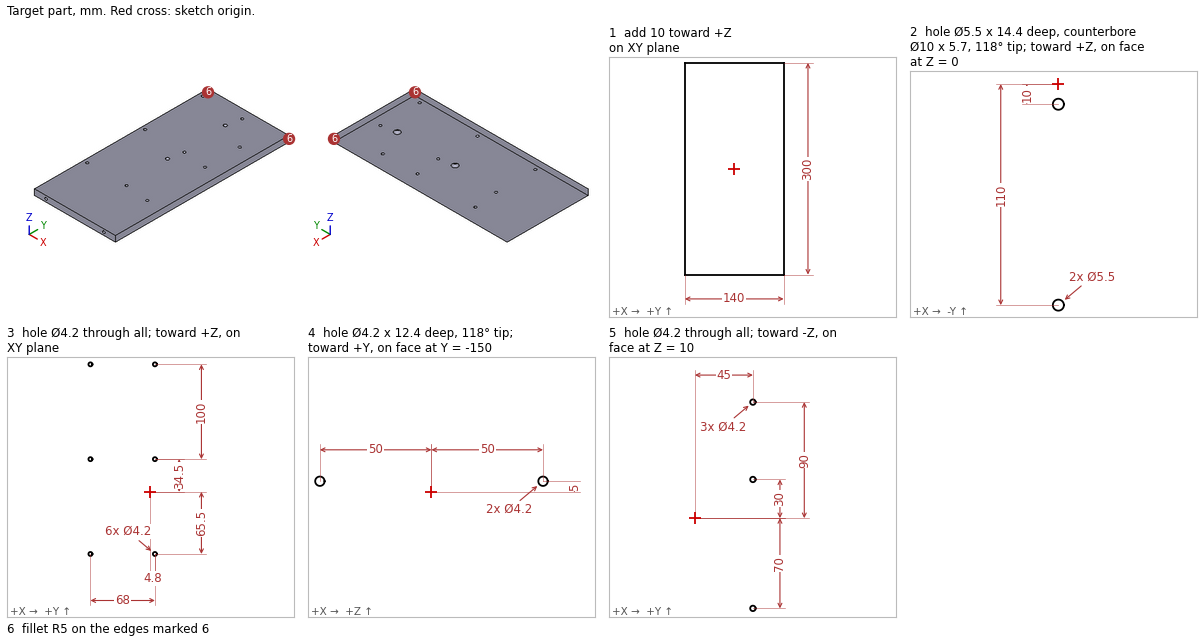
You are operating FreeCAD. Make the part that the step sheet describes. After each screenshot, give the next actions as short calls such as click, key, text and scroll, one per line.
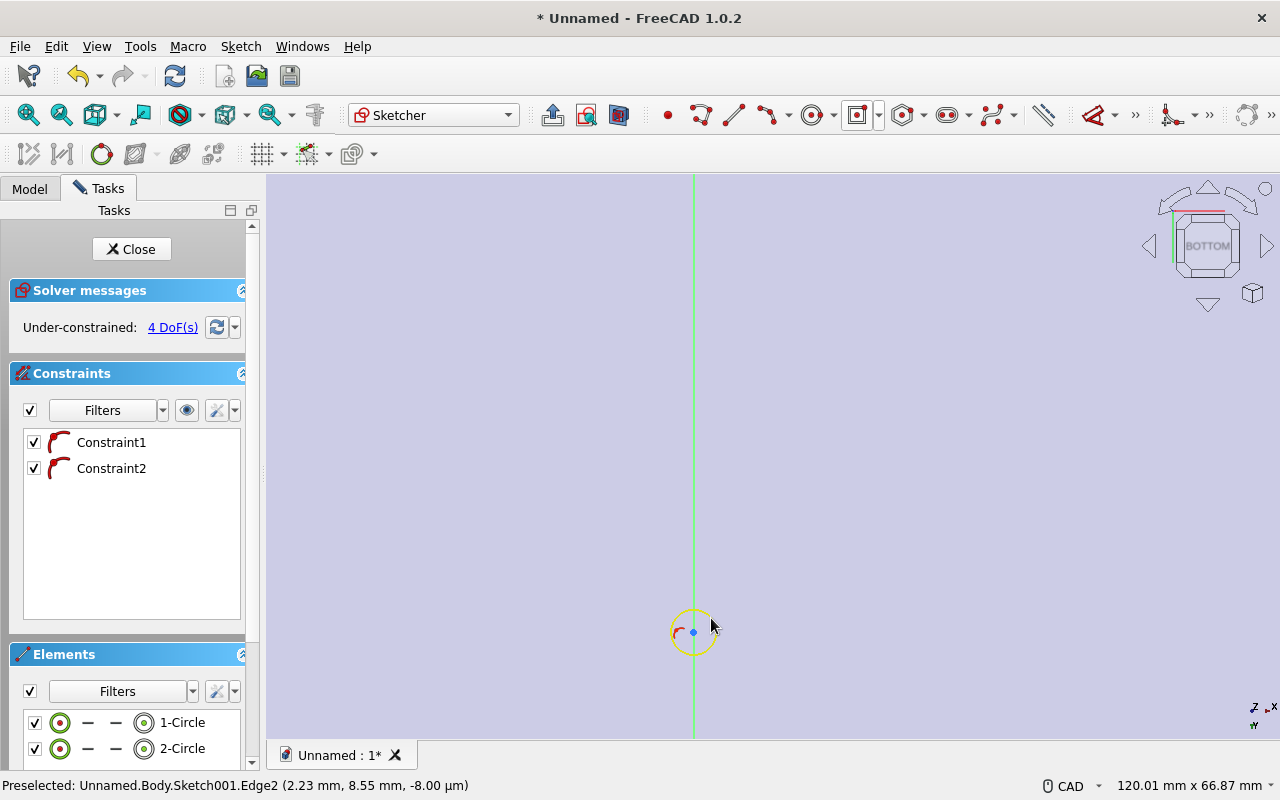
click(710, 616)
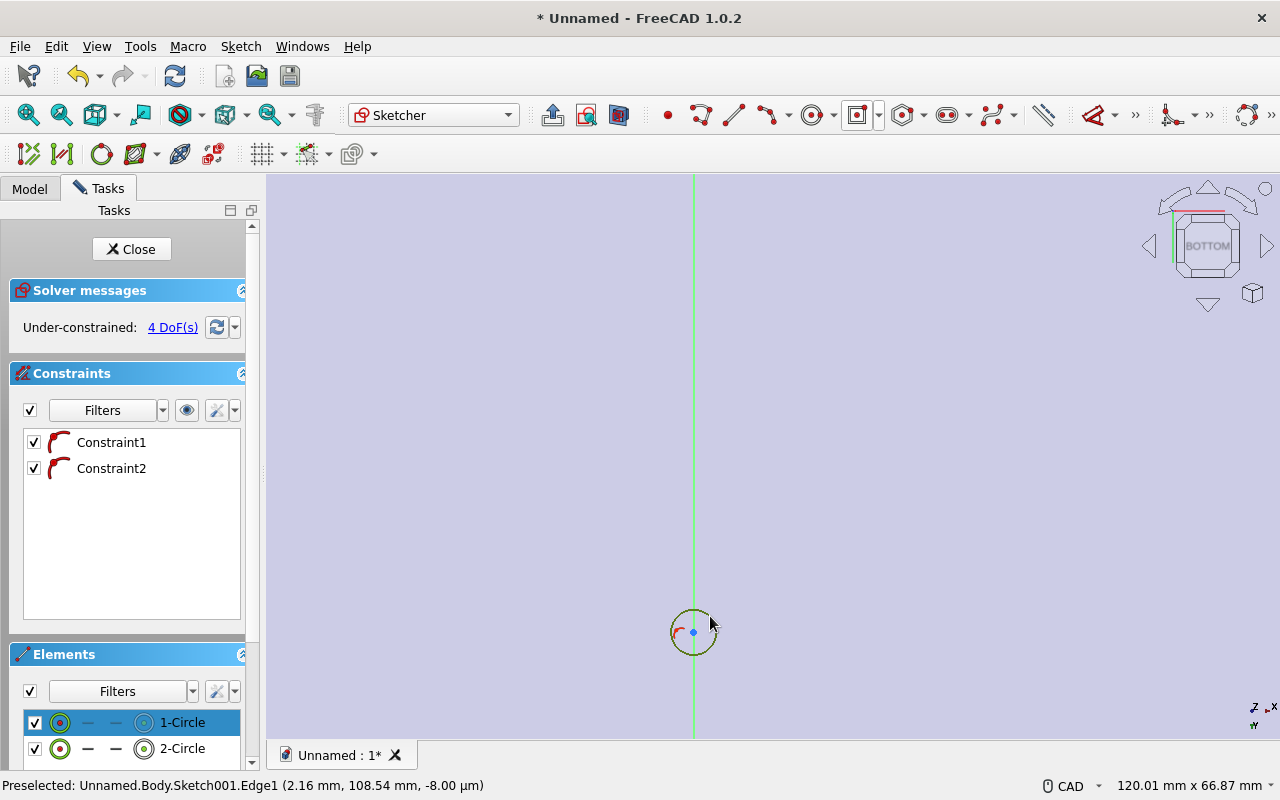
scroll(711, 618, down, 5)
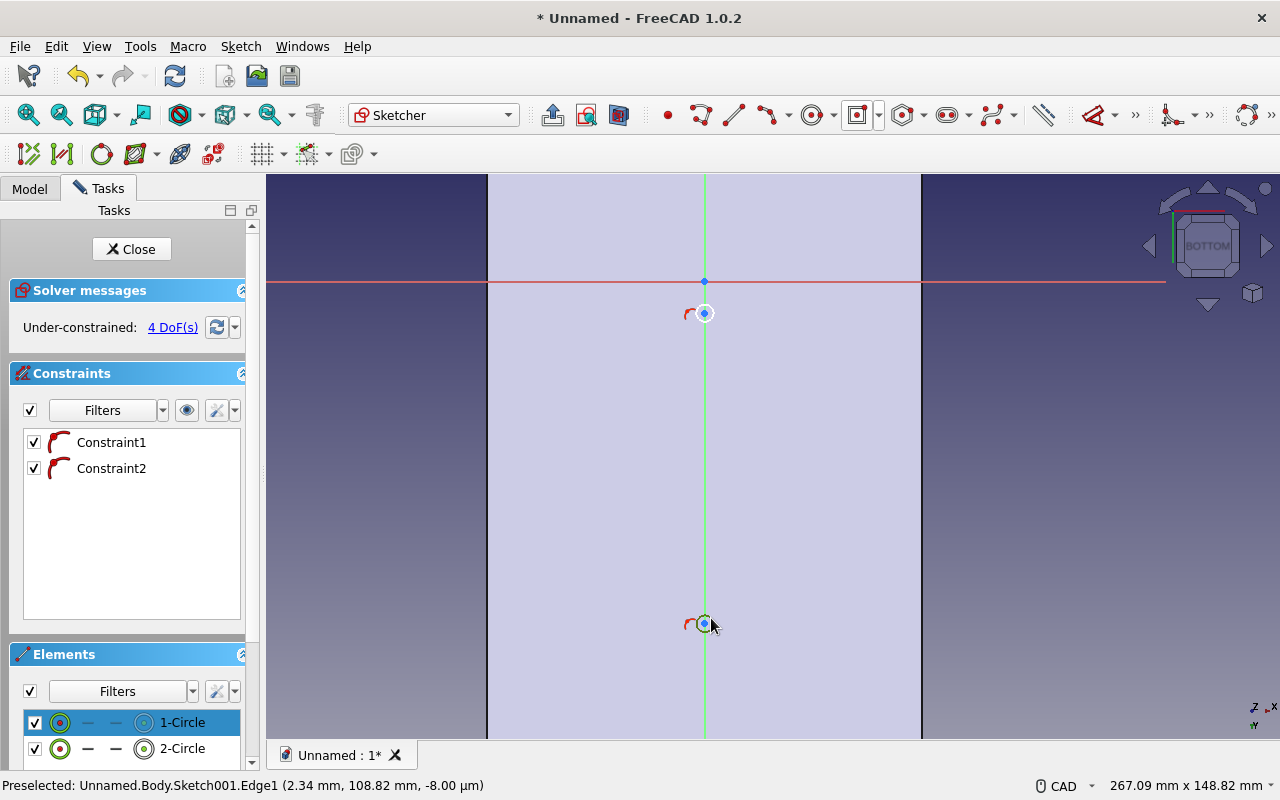
scroll(711, 307, up, 5)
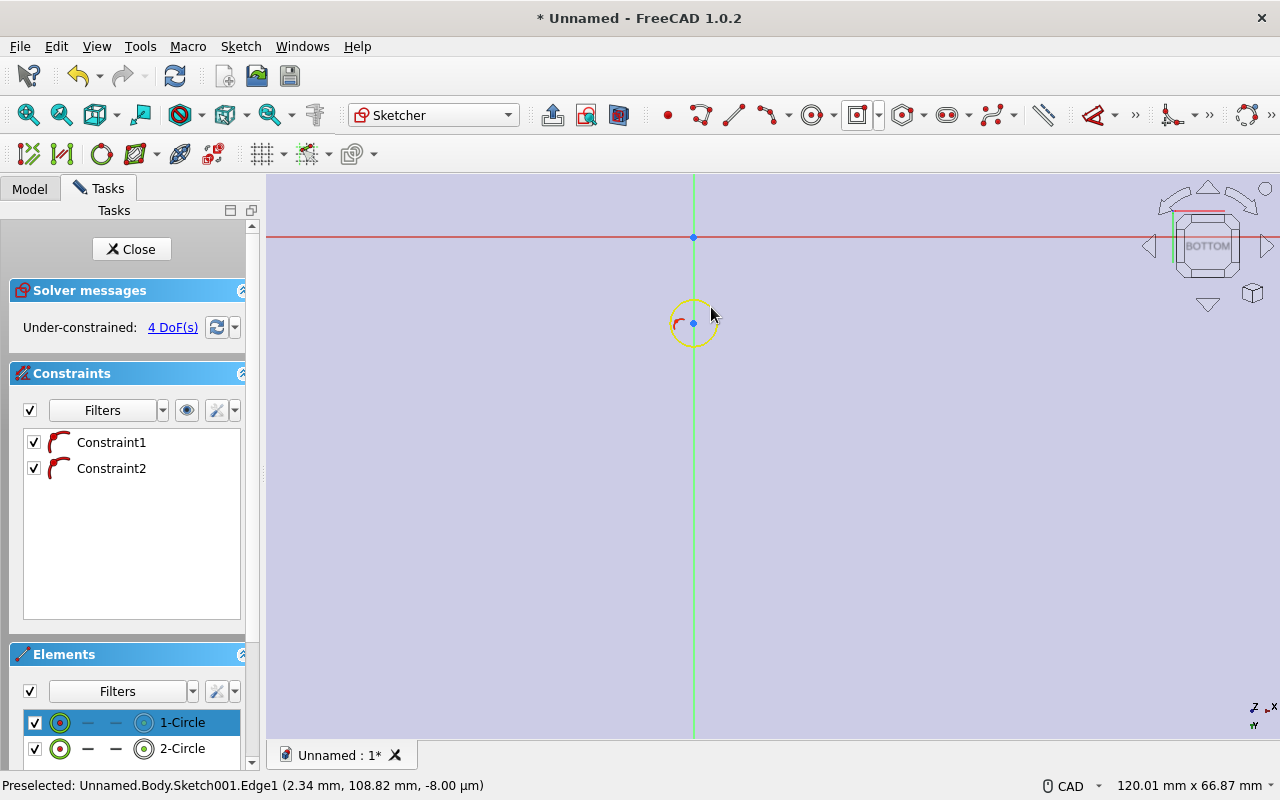
click(710, 307)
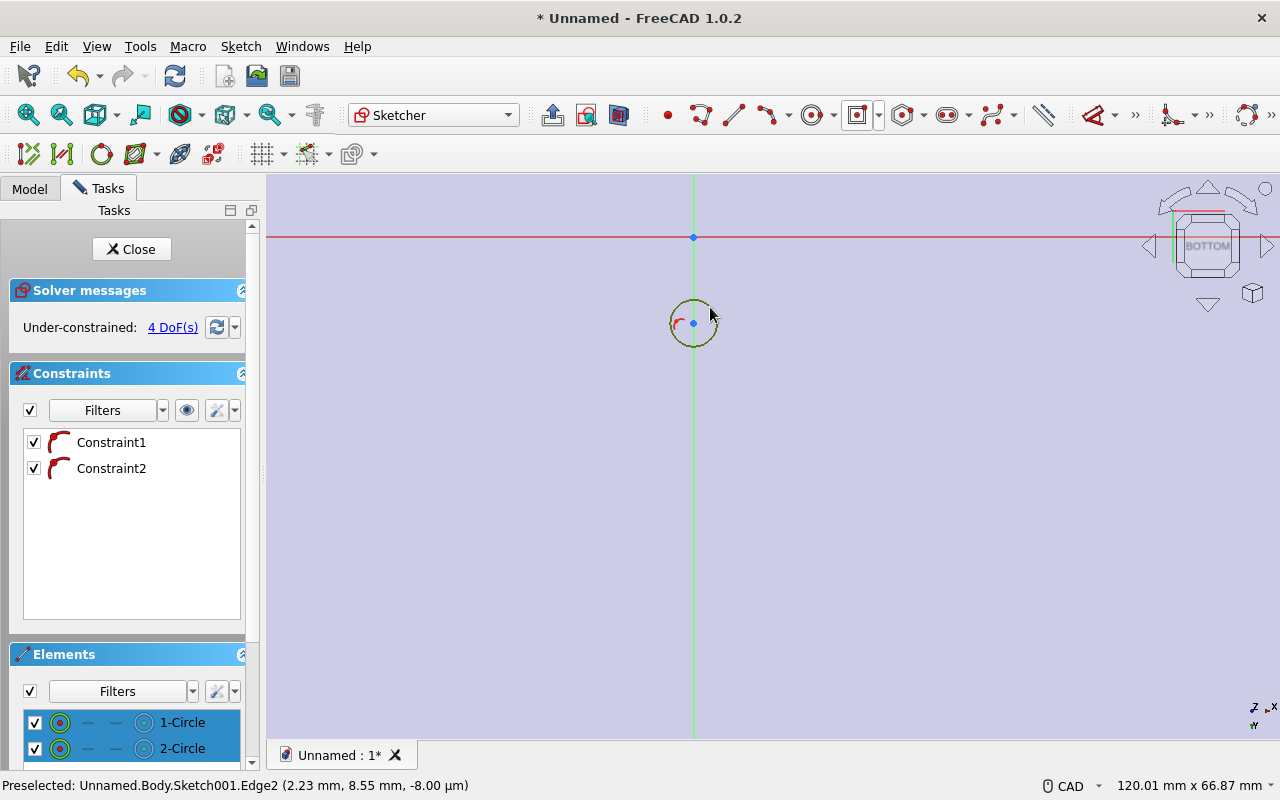
key(e)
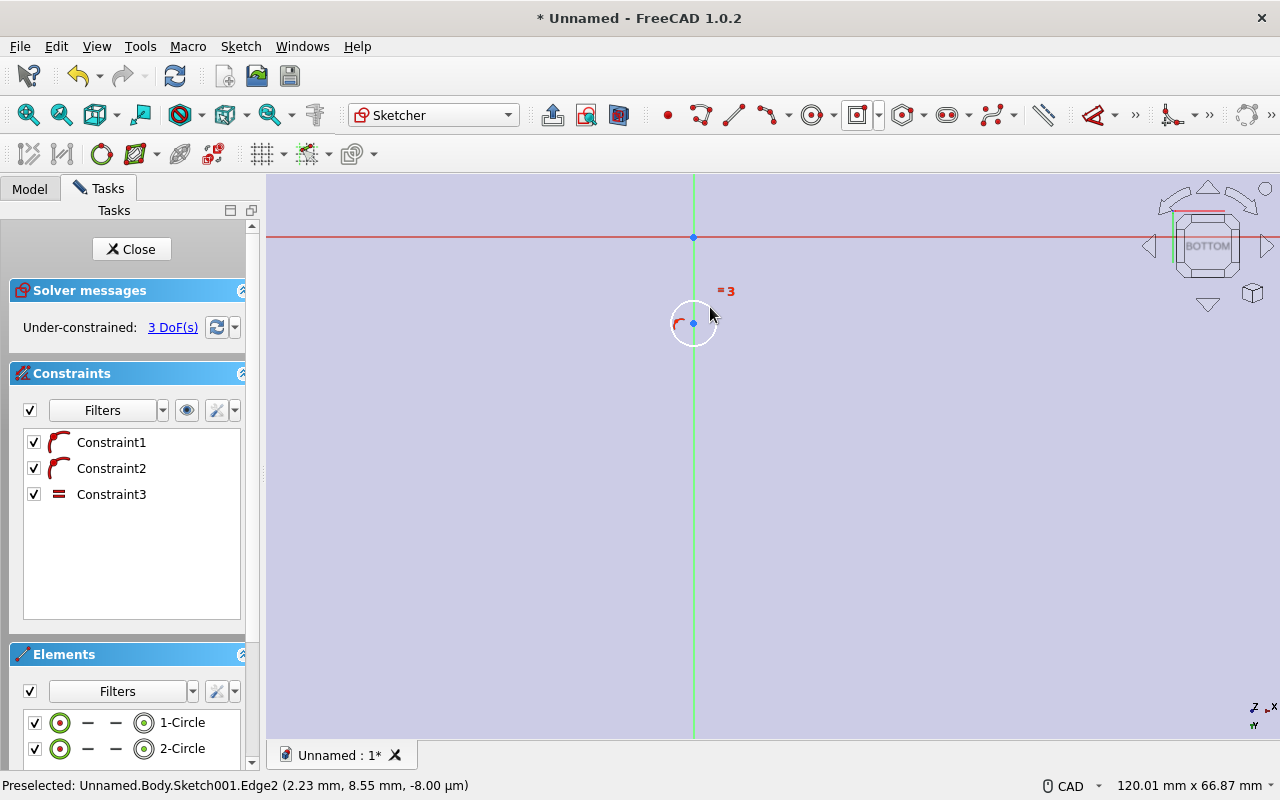
click(1092, 116)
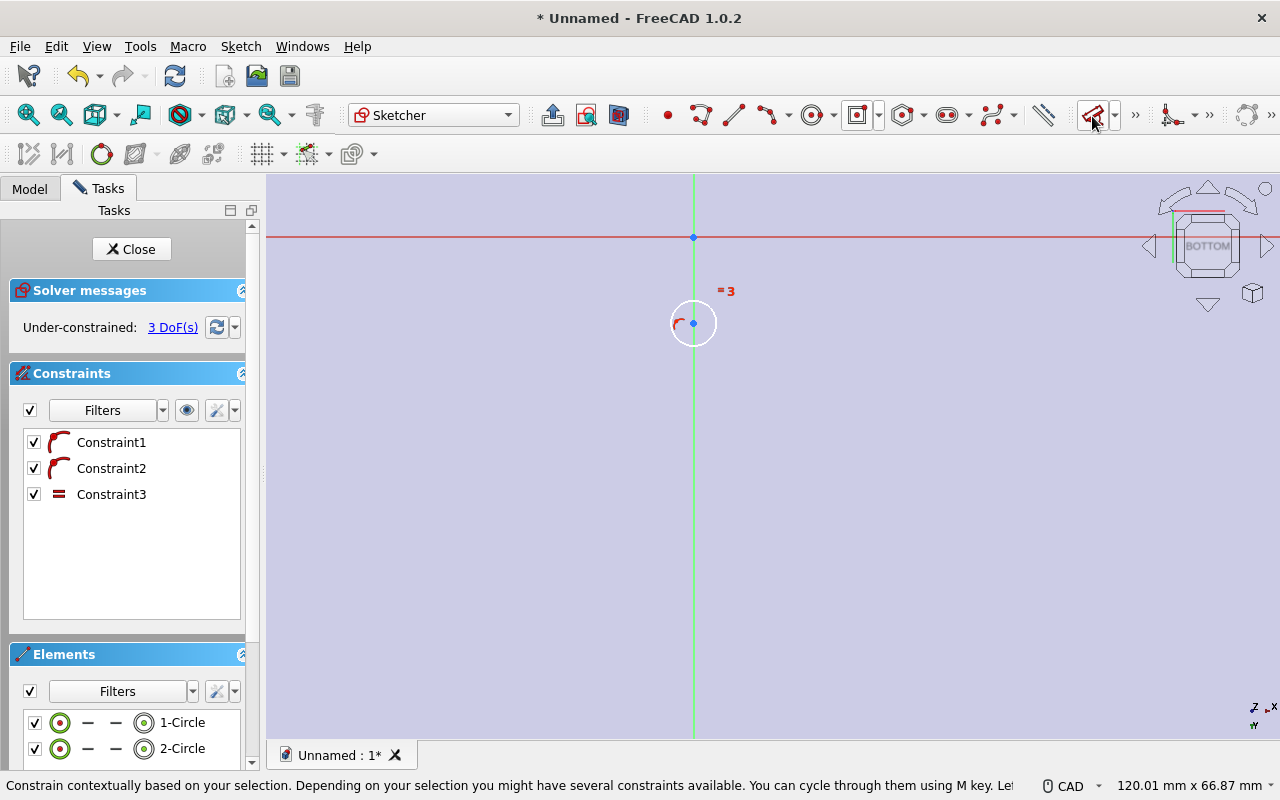
scroll(711, 307, down, 5)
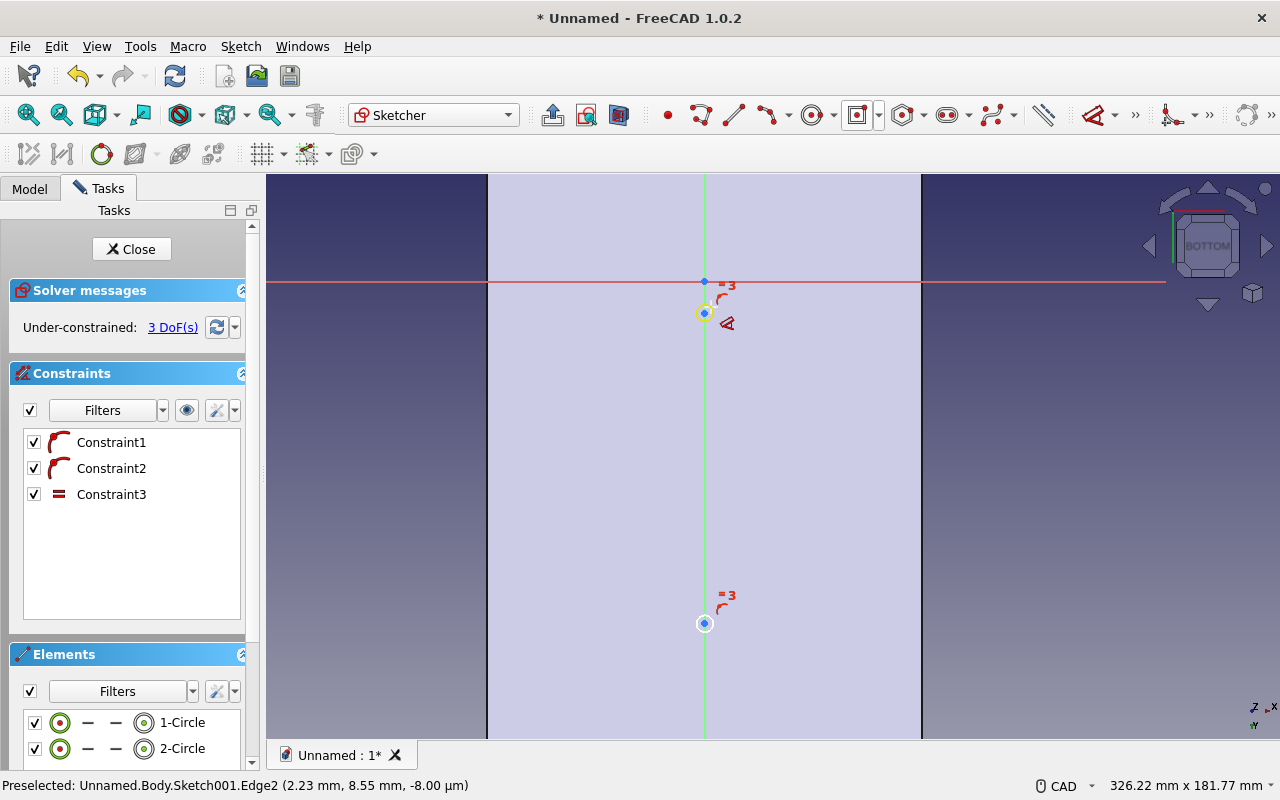
scroll(711, 618, up, 5)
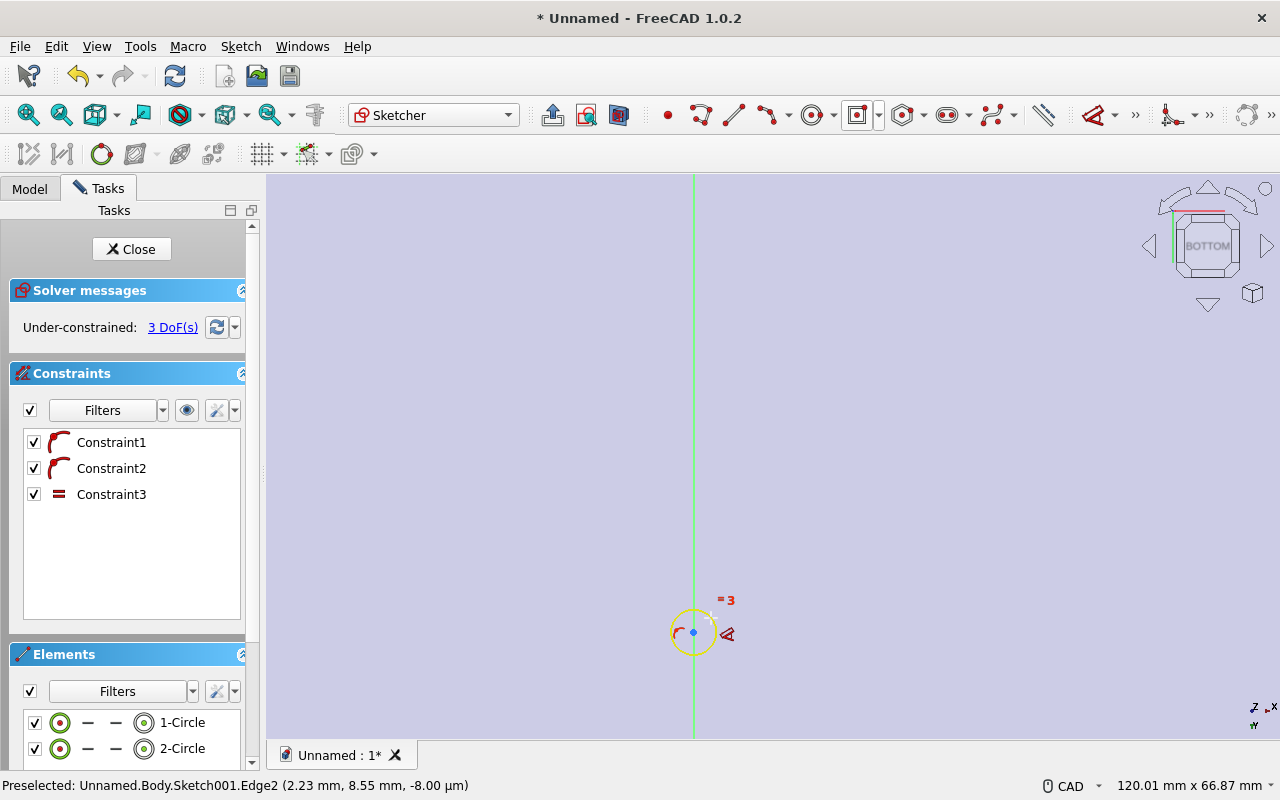
click(710, 616)
click(733, 593)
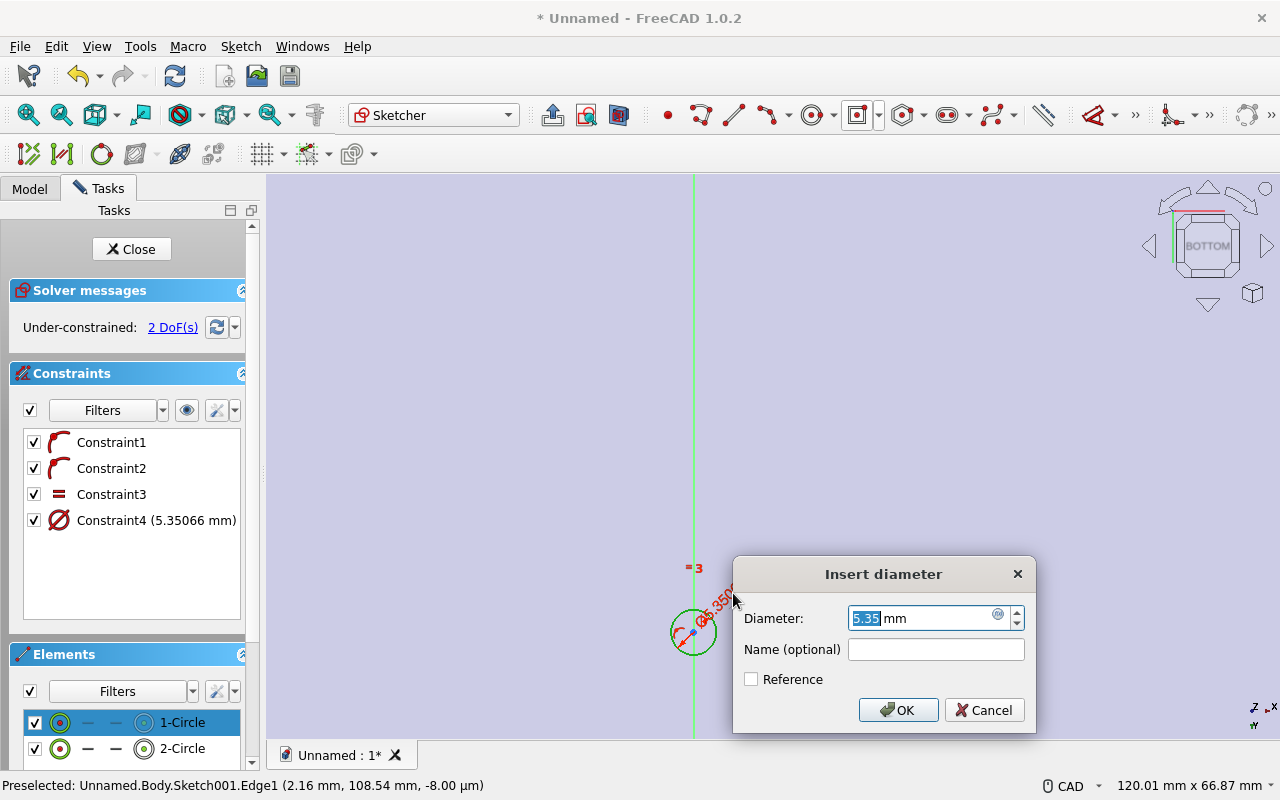
text(5.5)
key(Return)